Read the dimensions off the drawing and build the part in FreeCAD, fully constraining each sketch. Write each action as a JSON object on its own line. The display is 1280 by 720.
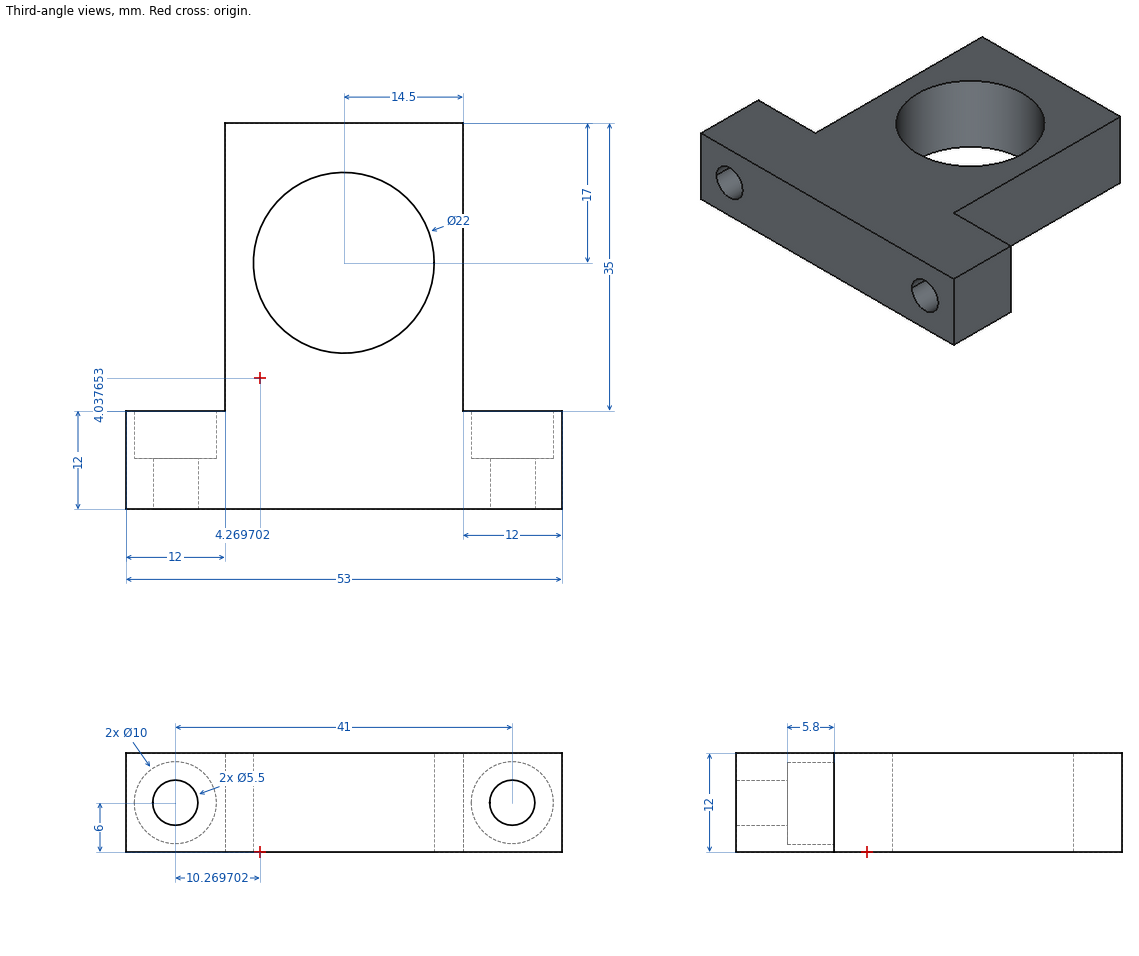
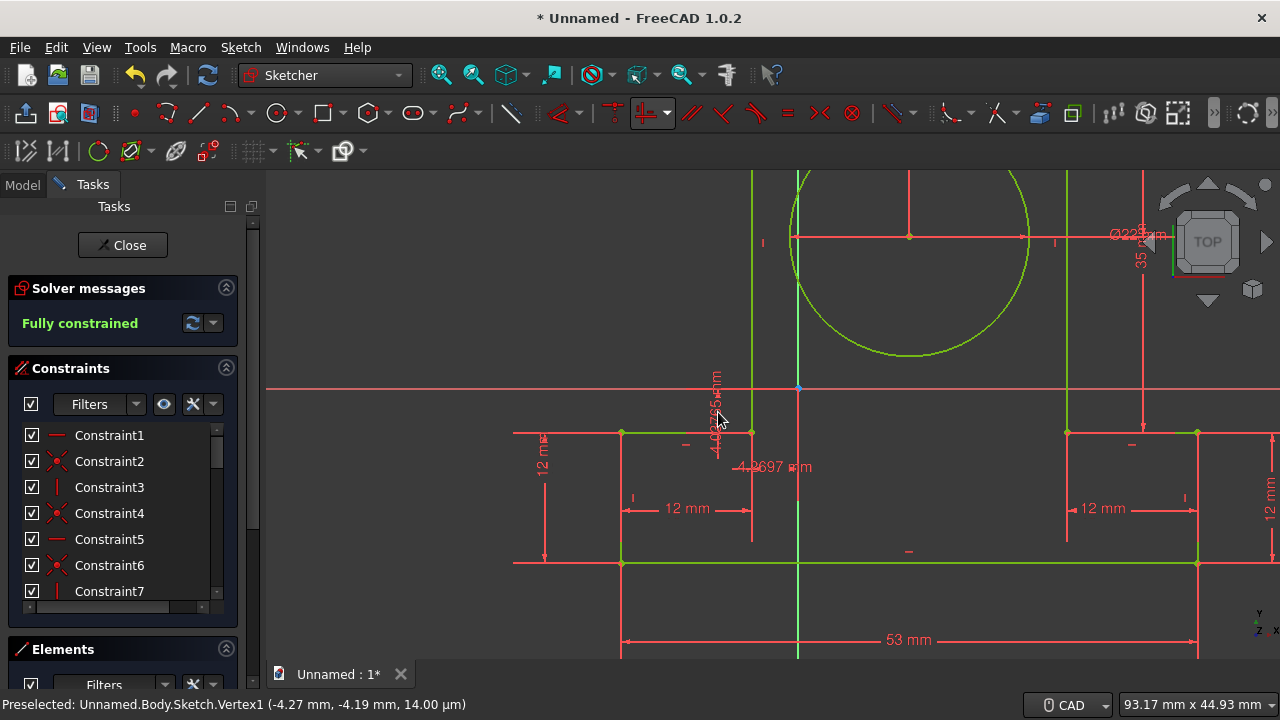
{"action": "left_click", "coordinate": [123, 245]}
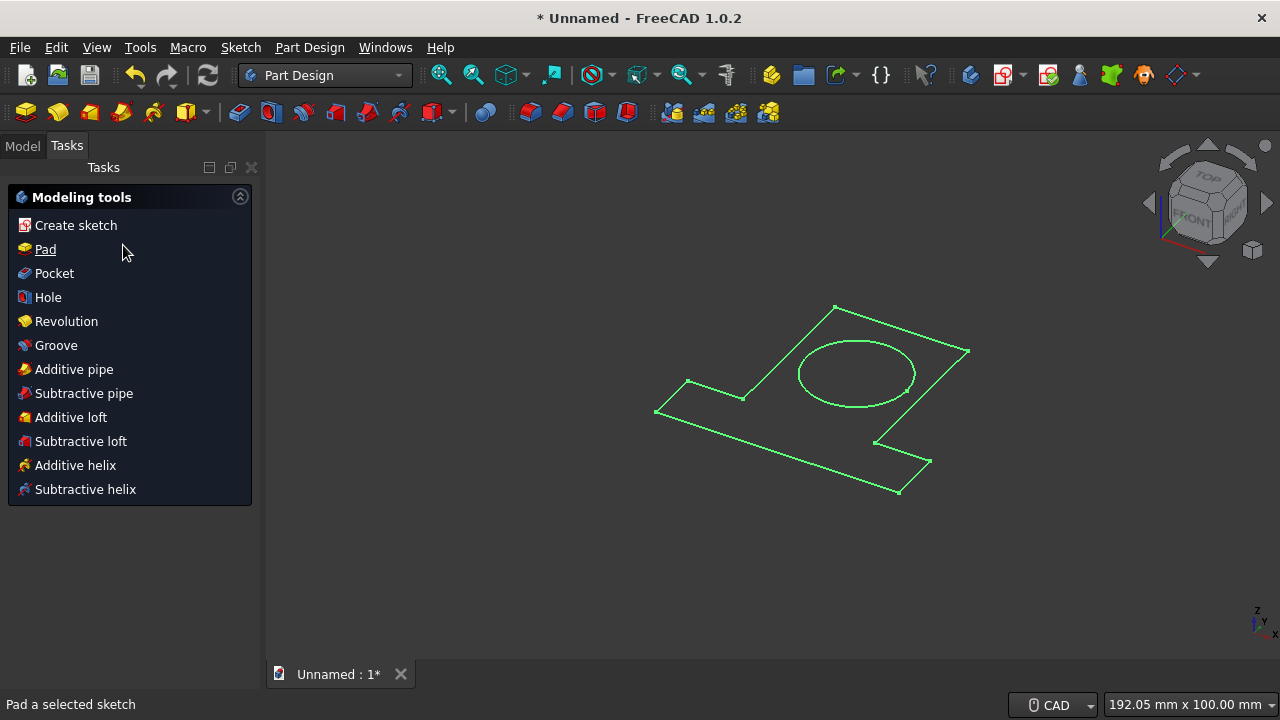
{"action": "left_click", "coordinate": [26, 112]}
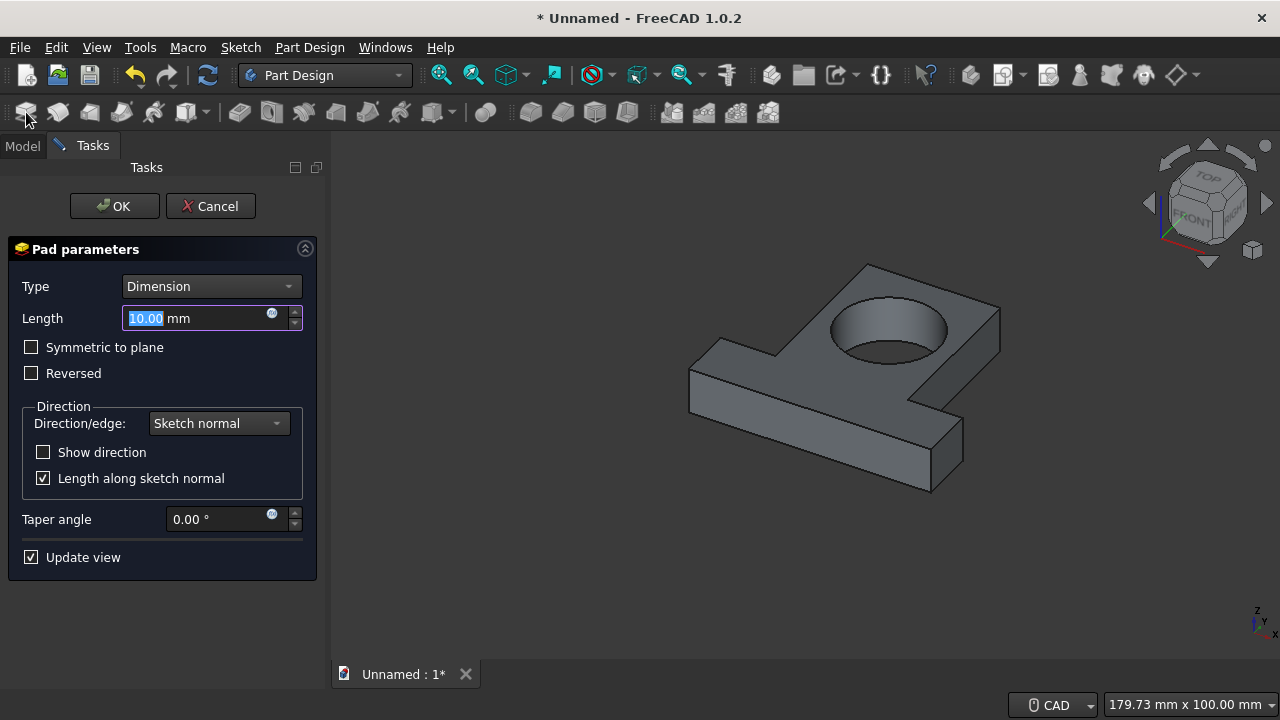
{"action": "type", "text": "12"}
{"action": "key", "text": "Tab"}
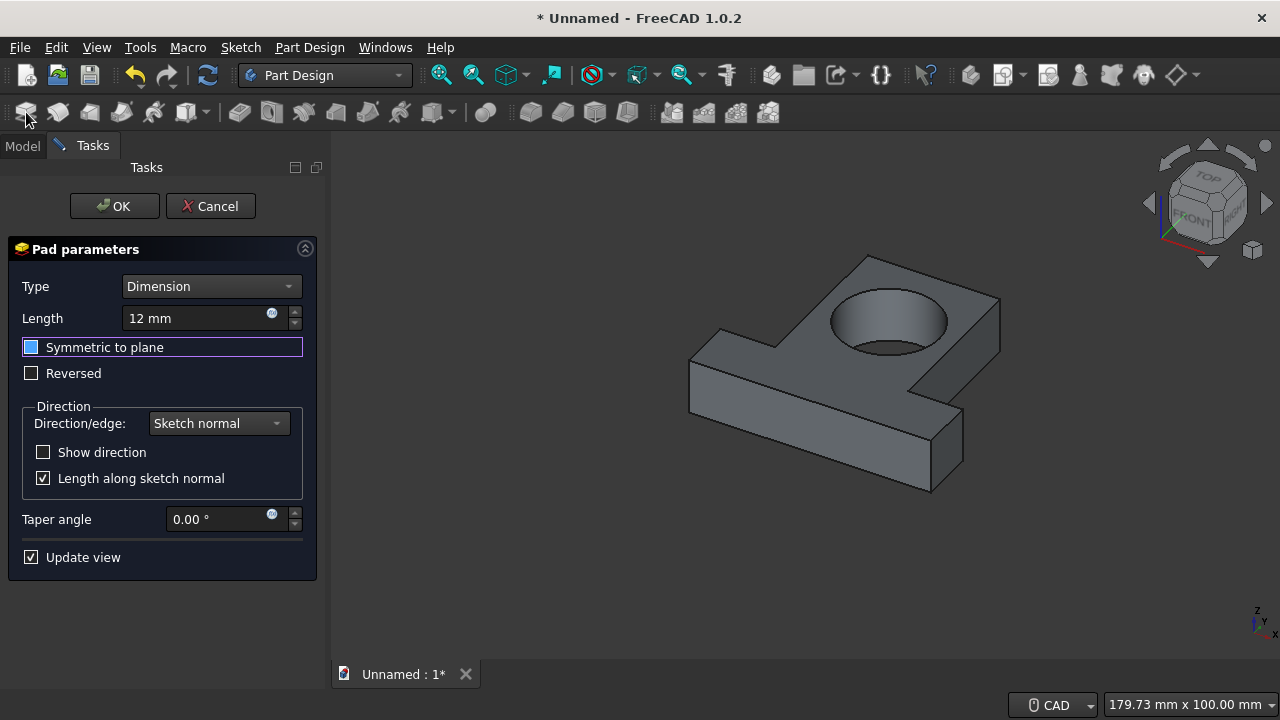
{"action": "left_click", "coordinate": [115, 206]}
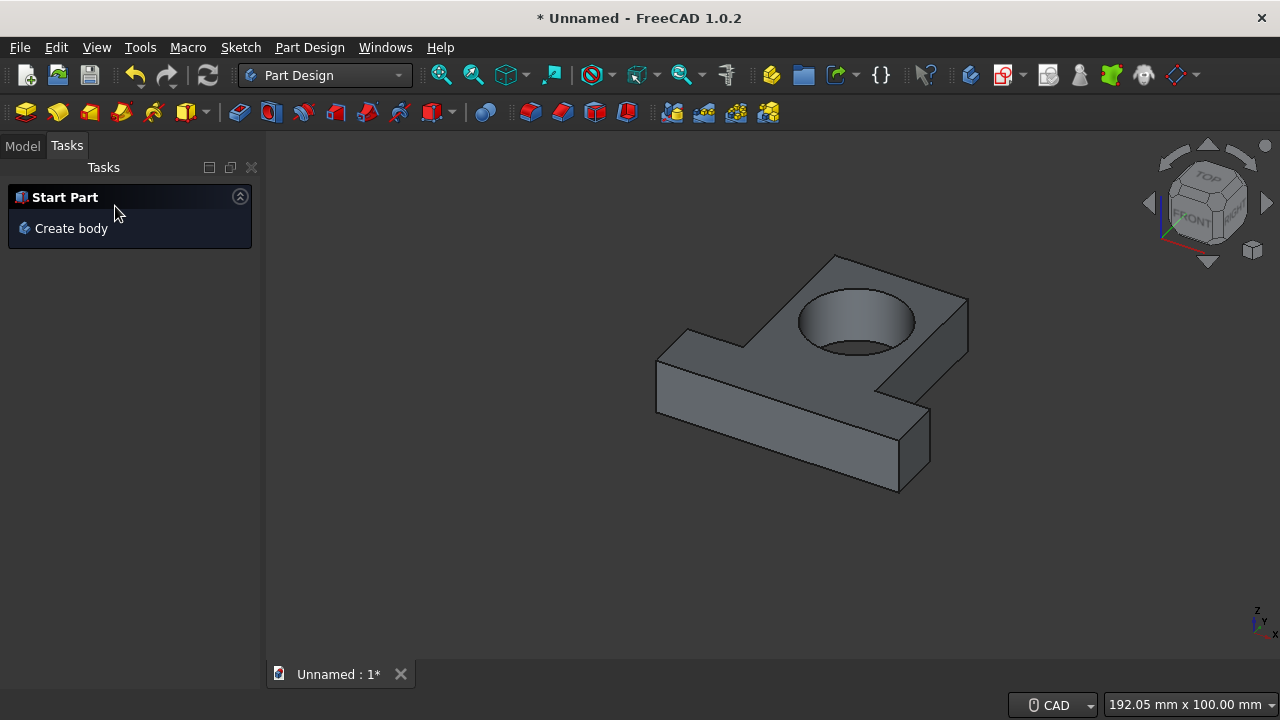
{"action": "key", "text": "4"}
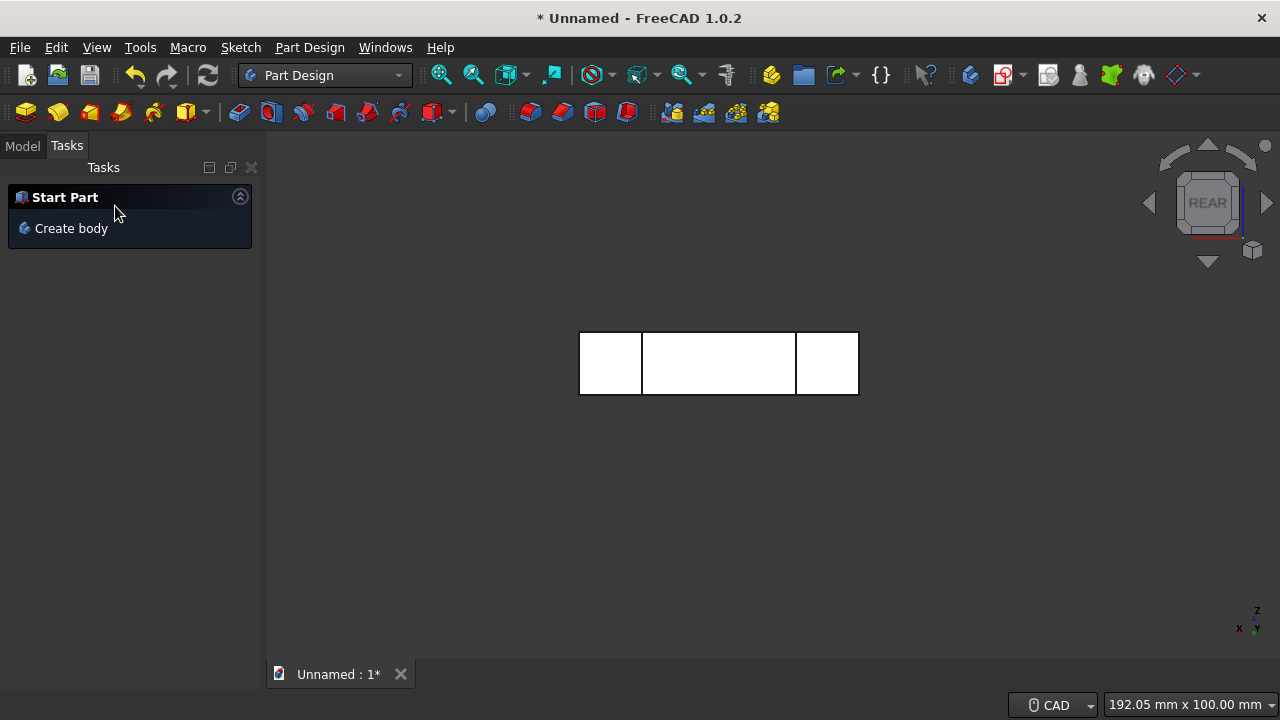
{"action": "left_click", "coordinate": [442, 76]}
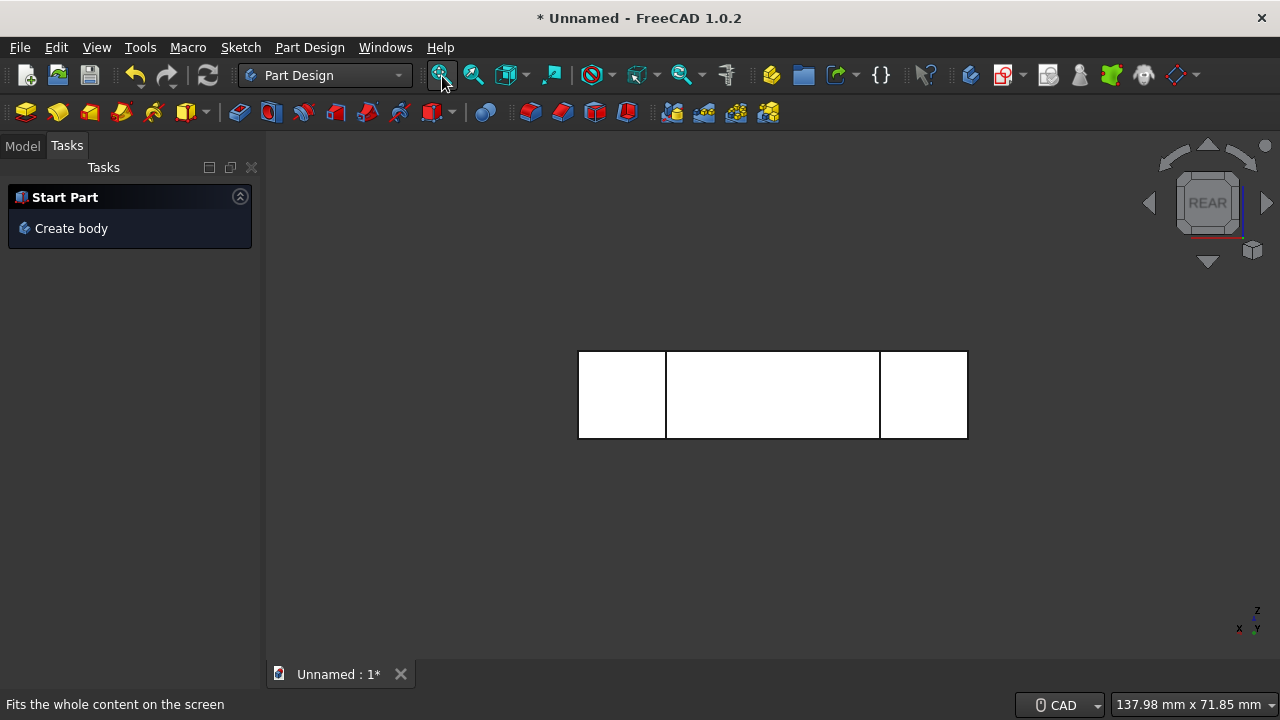
{"action": "left_click", "coordinate": [622, 394]}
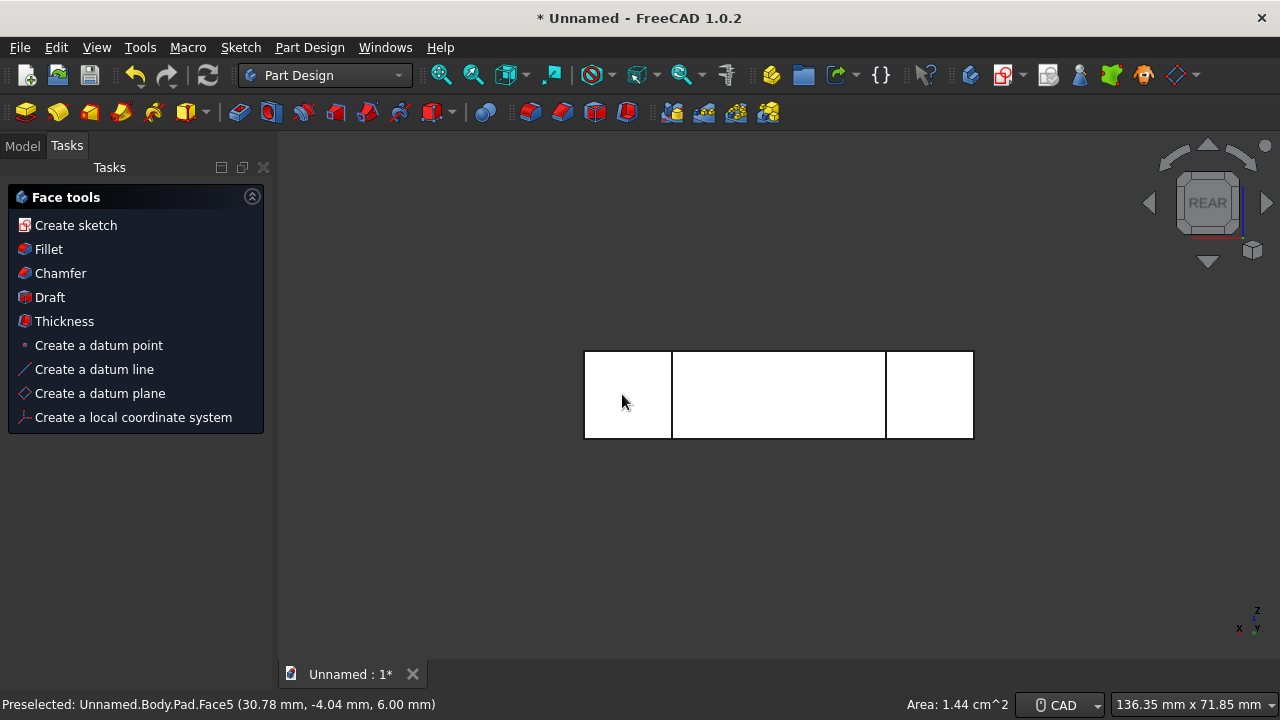
{"action": "left_click", "coordinate": [1004, 76]}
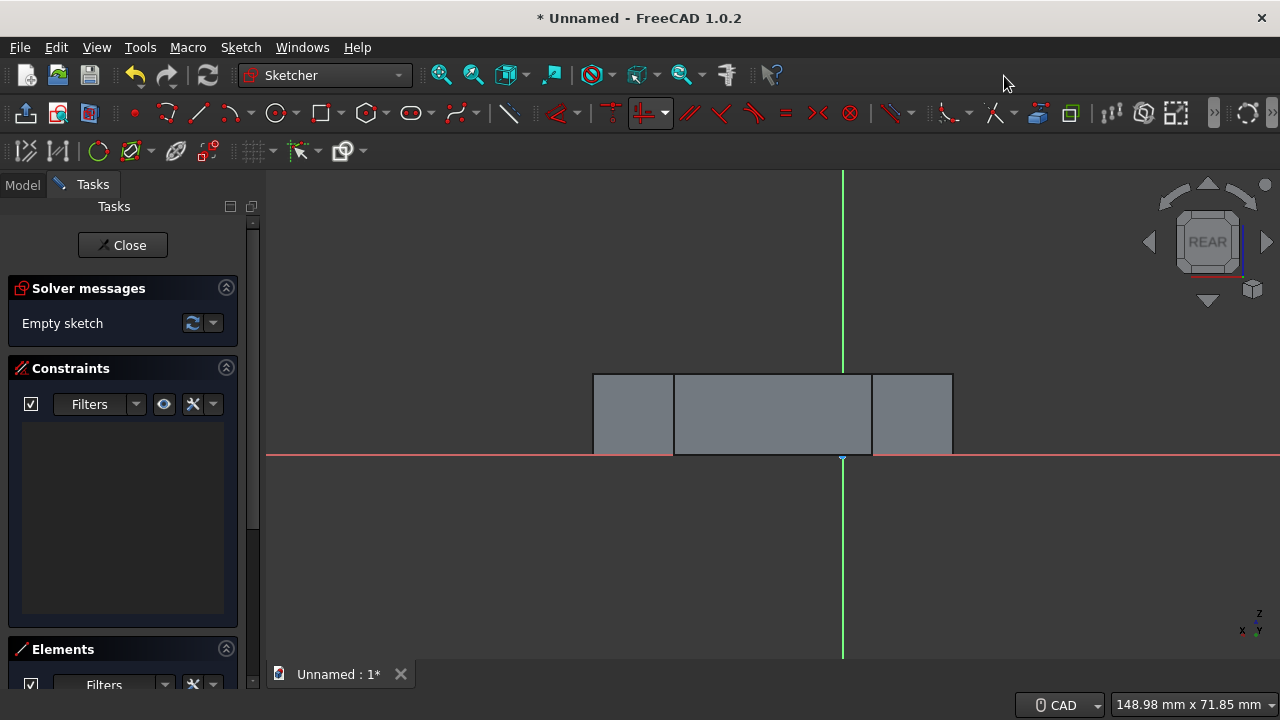
{"action": "left_click", "coordinate": [90, 114]}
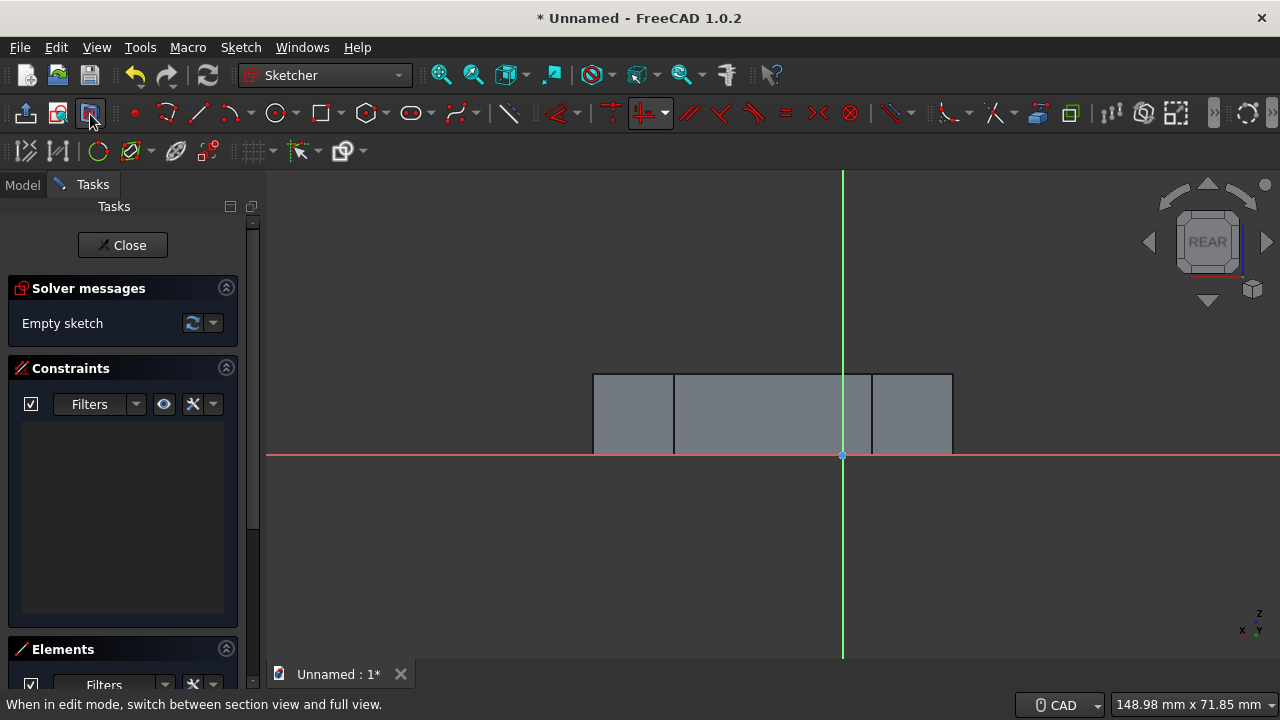
{"action": "scroll", "coordinate": [856, 439], "scroll_direction": "up", "scroll_amount": 3}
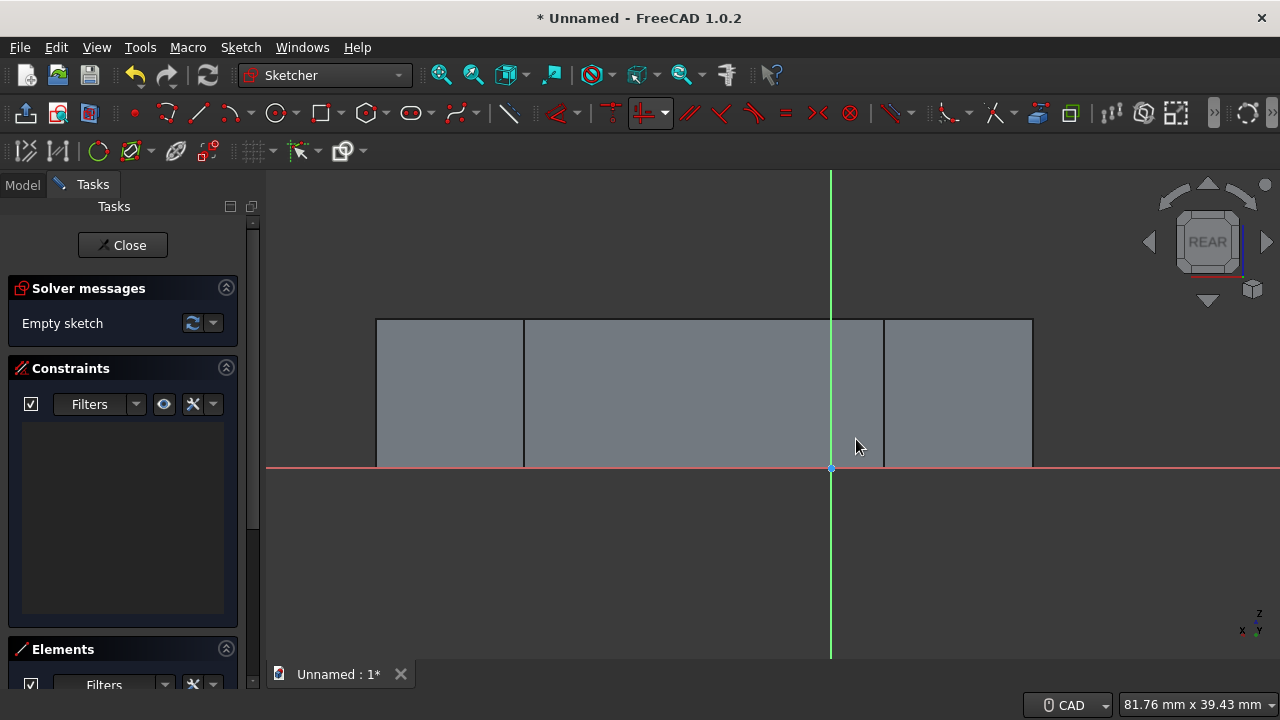
{"action": "left_click", "coordinate": [276, 114]}